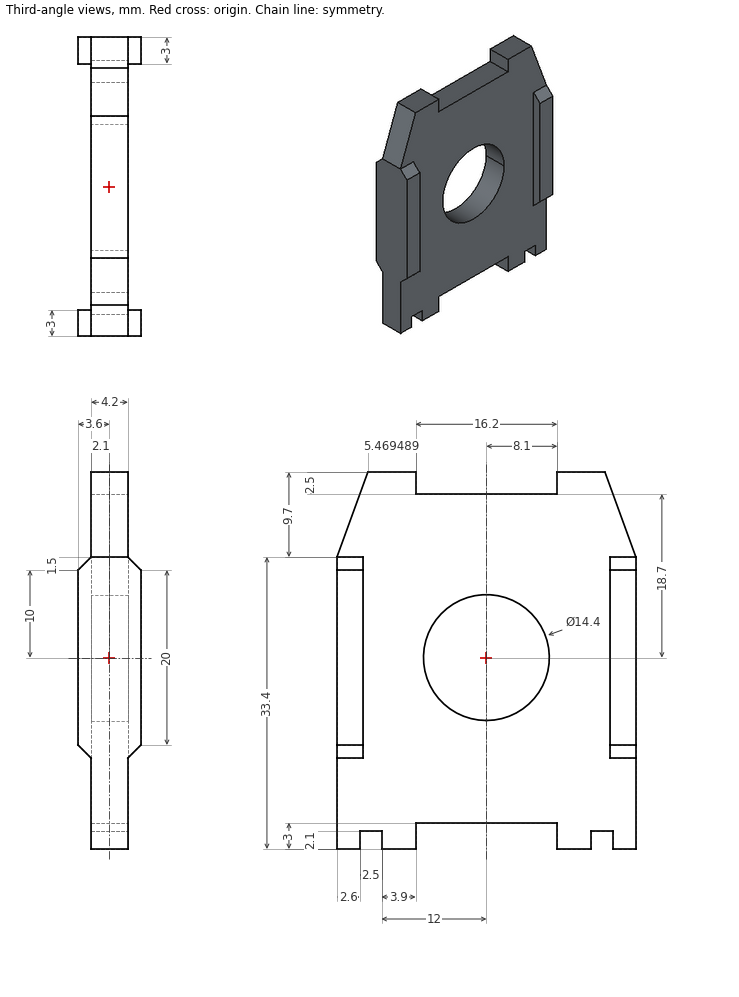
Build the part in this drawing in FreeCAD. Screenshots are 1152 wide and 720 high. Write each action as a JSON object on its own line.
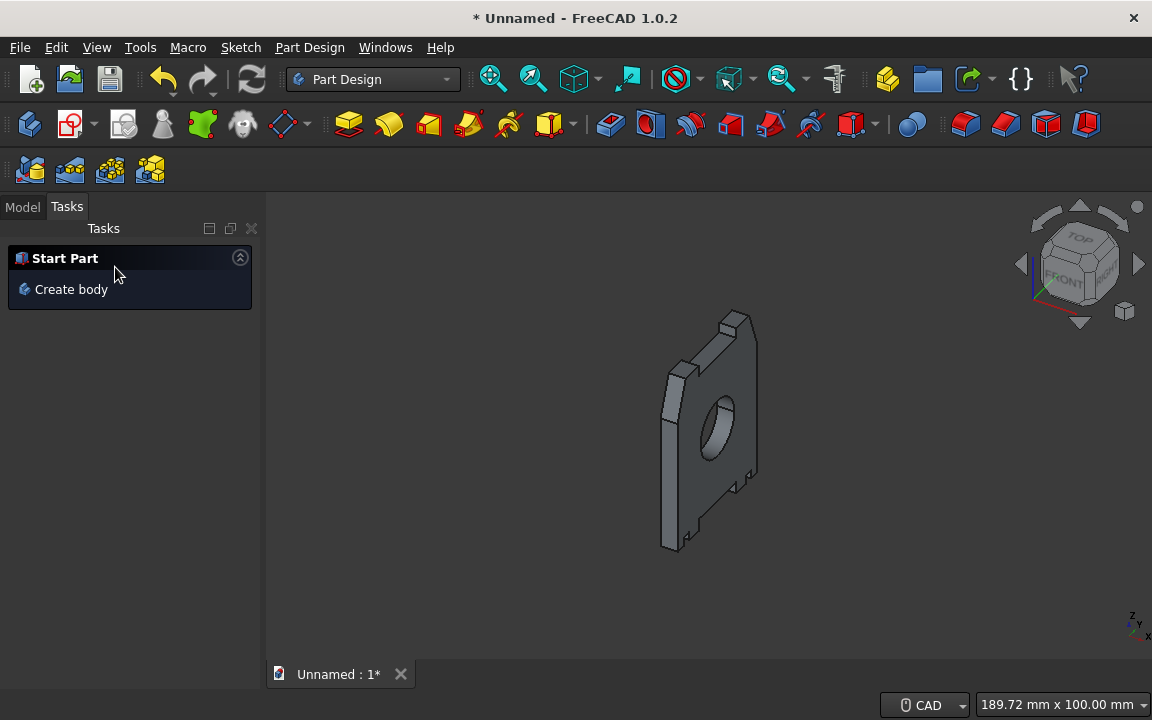
{"action": "key", "text": "4"}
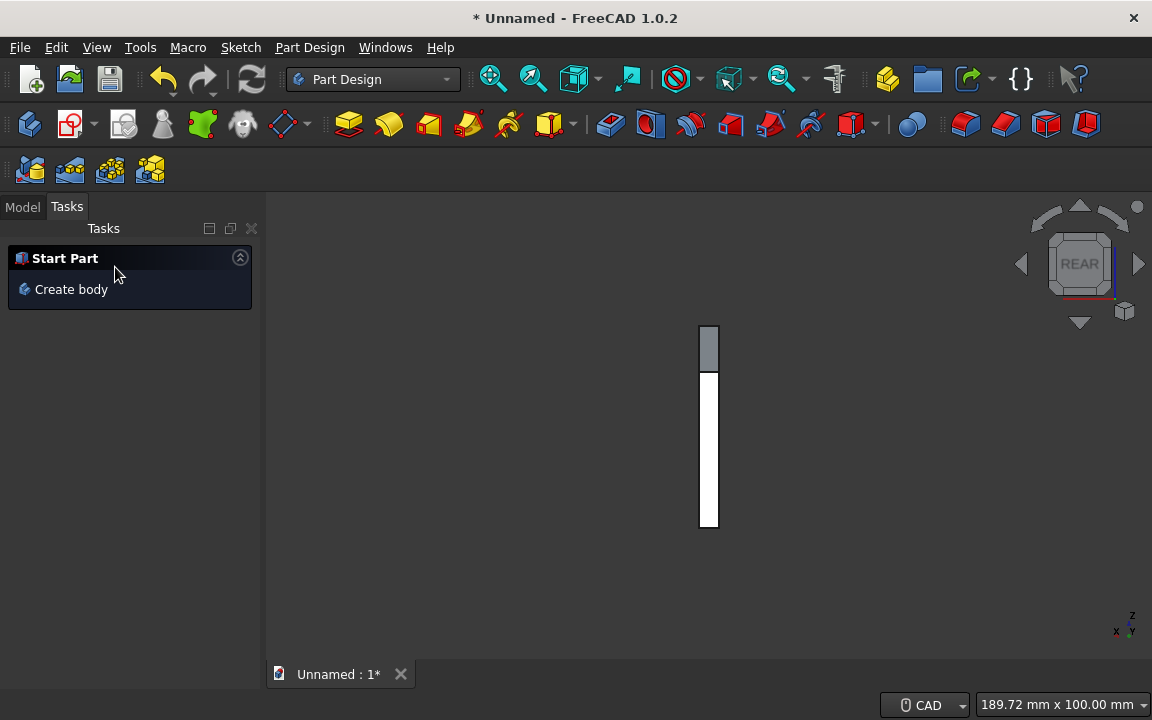
{"action": "key", "text": "v f"}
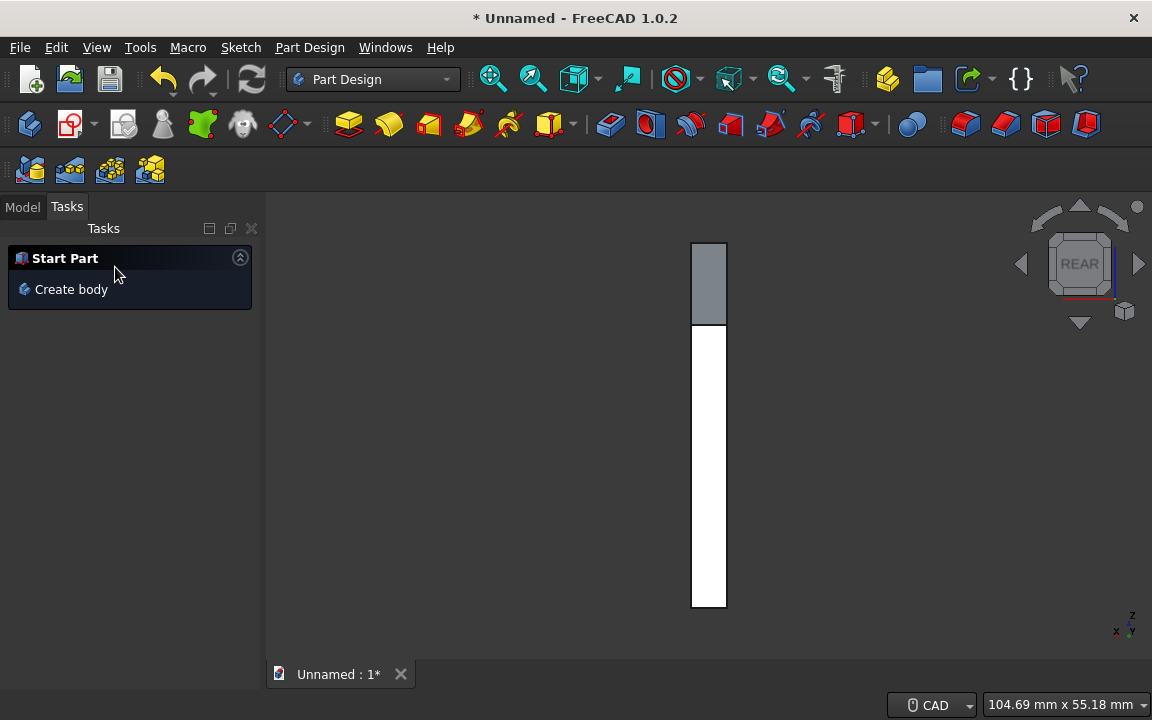
{"action": "left_click", "coordinate": [709, 546]}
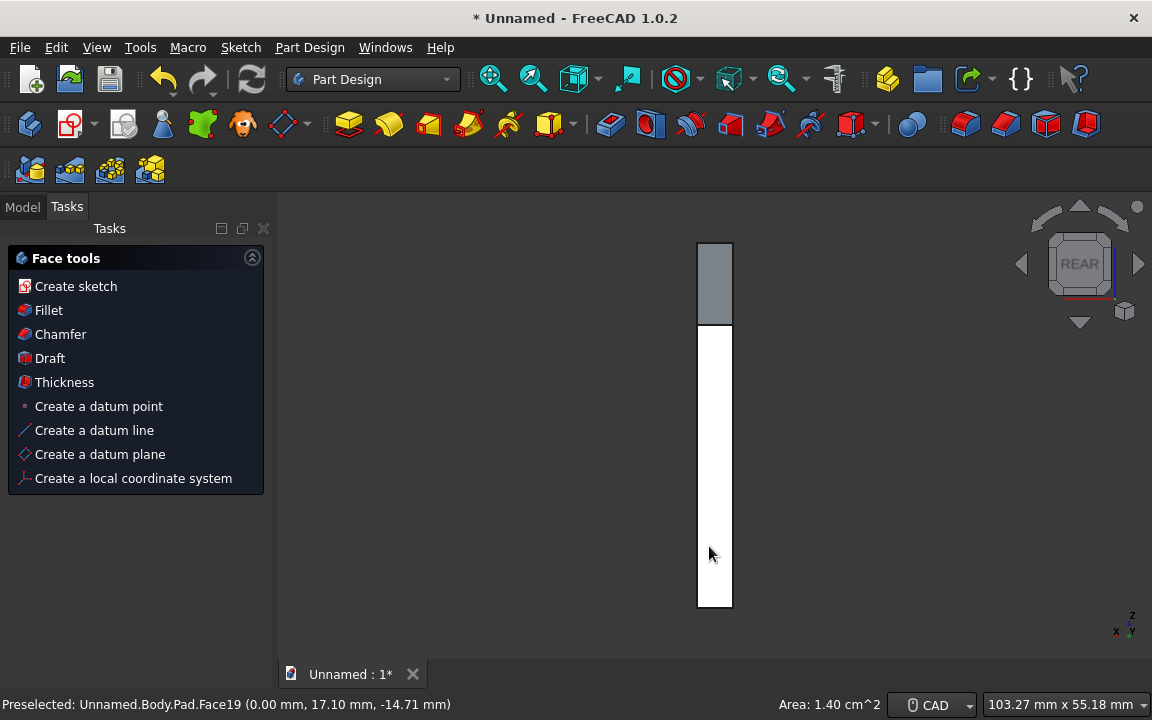
{"action": "left_click", "coordinate": [70, 124]}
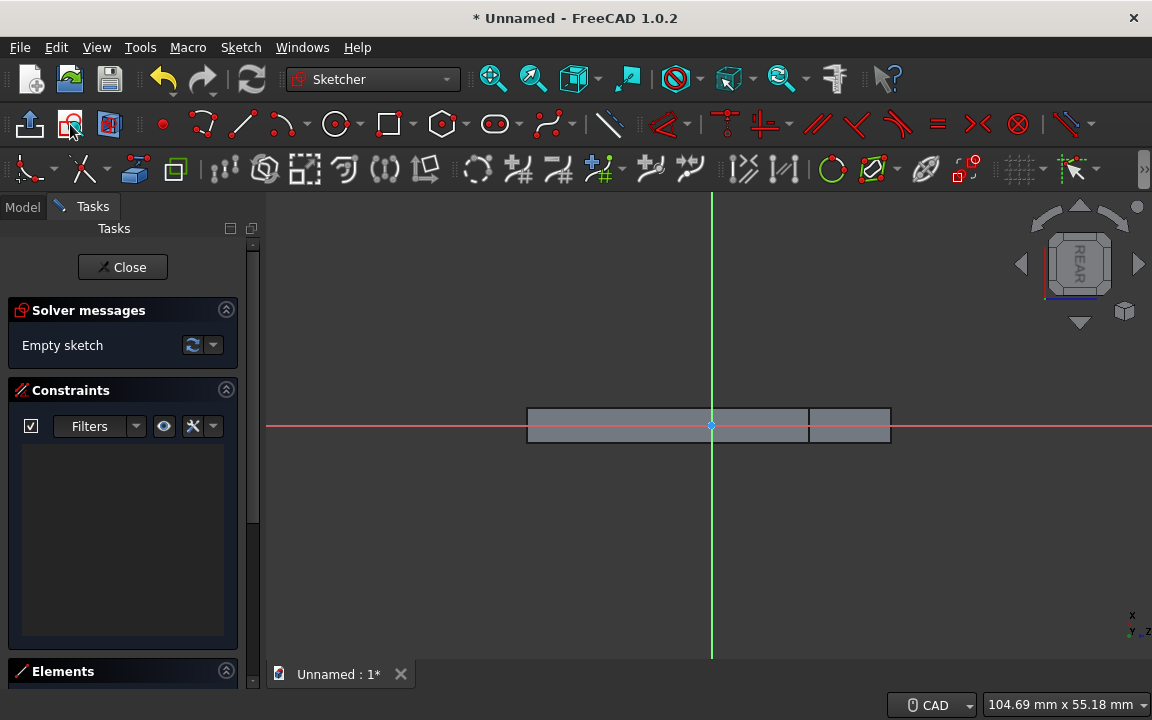
{"action": "scroll", "coordinate": [754, 425], "scroll_direction": "up", "scroll_amount": 5}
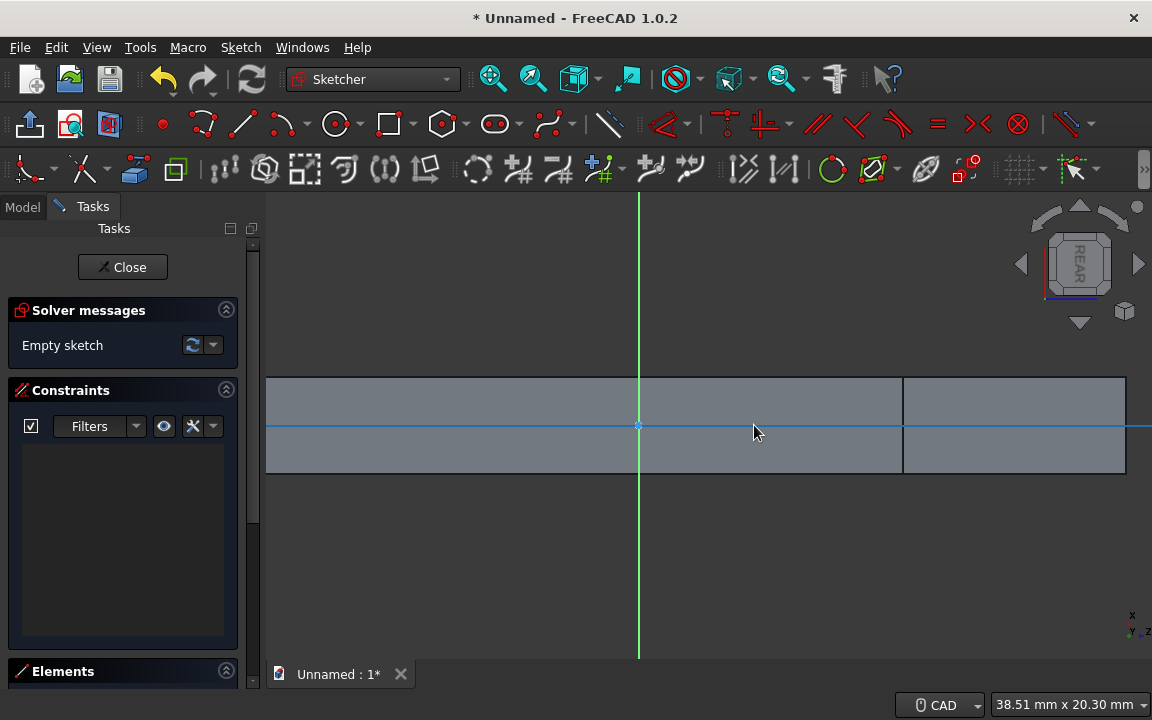
{"action": "key", "text": "g m"}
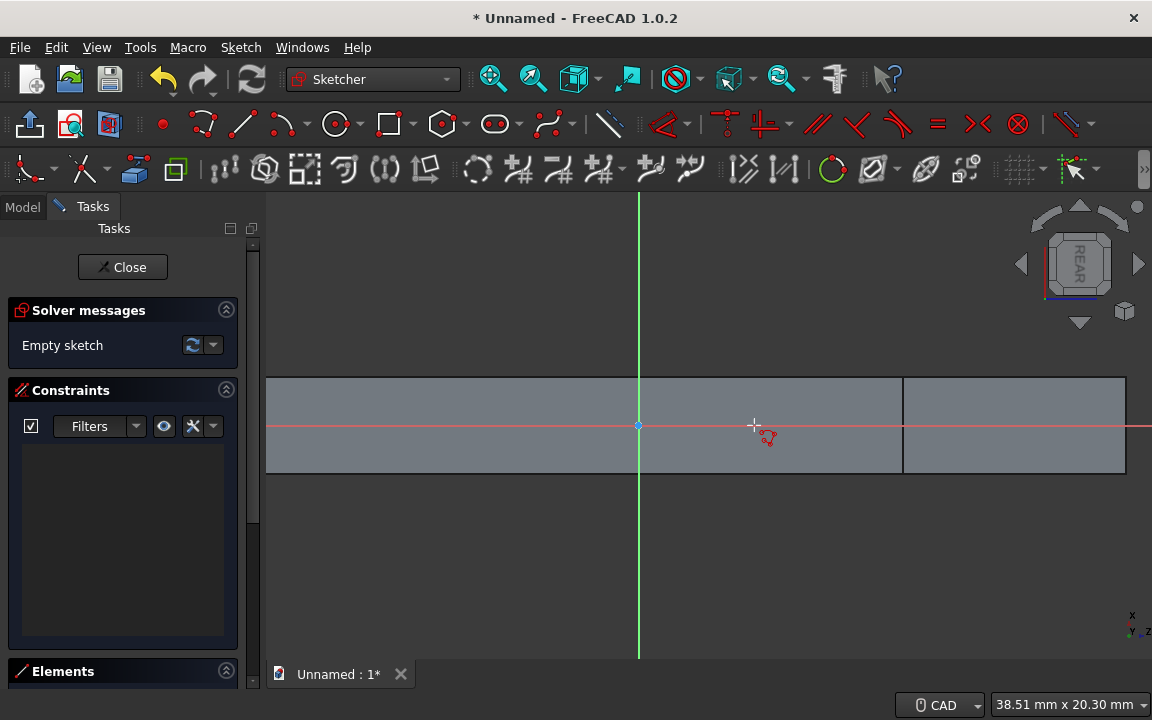
{"action": "left_click", "coordinate": [869, 508]}
{"action": "left_click", "coordinate": [903, 474]}
{"action": "left_click", "coordinate": [903, 377]}
{"action": "left_click", "coordinate": [869, 343]}
{"action": "left_click", "coordinate": [409, 343]}
{"action": "left_click", "coordinate": [374, 377]}
{"action": "left_click", "coordinate": [374, 474]}
{"action": "left_click", "coordinate": [409, 508]}
{"action": "left_click", "coordinate": [869, 509]}
{"action": "key", "text": "Escape"}
{"action": "key", "text": "Escape"}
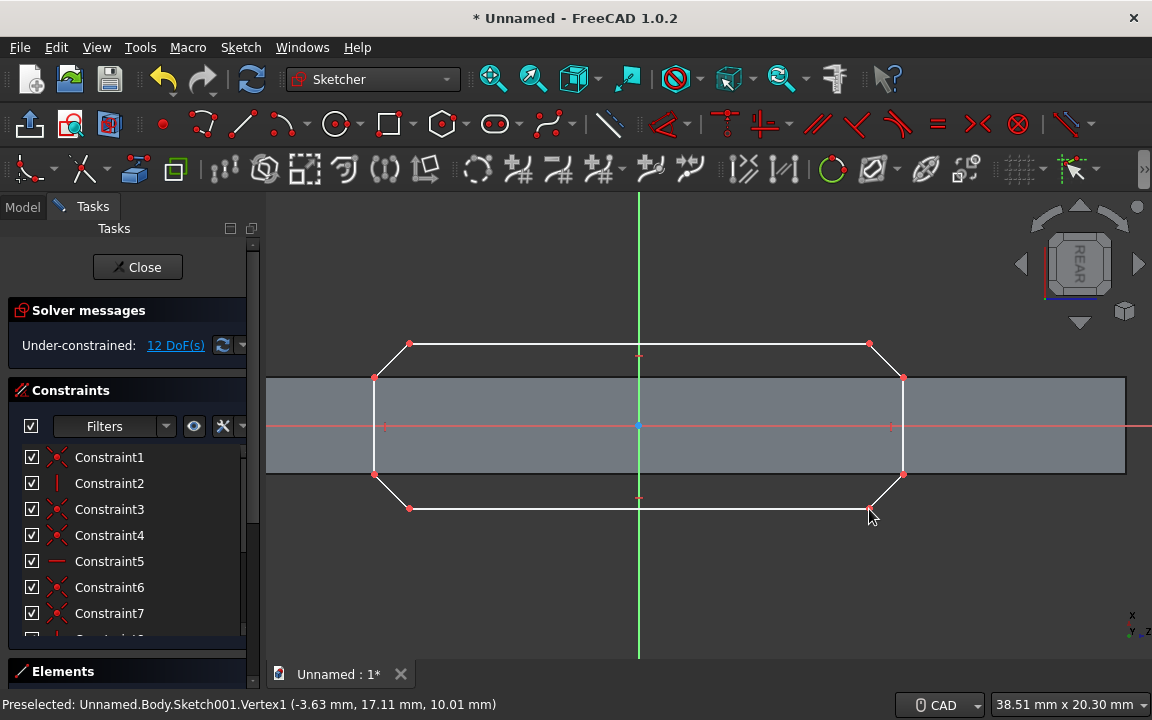
{"action": "left_click", "coordinate": [869, 509]}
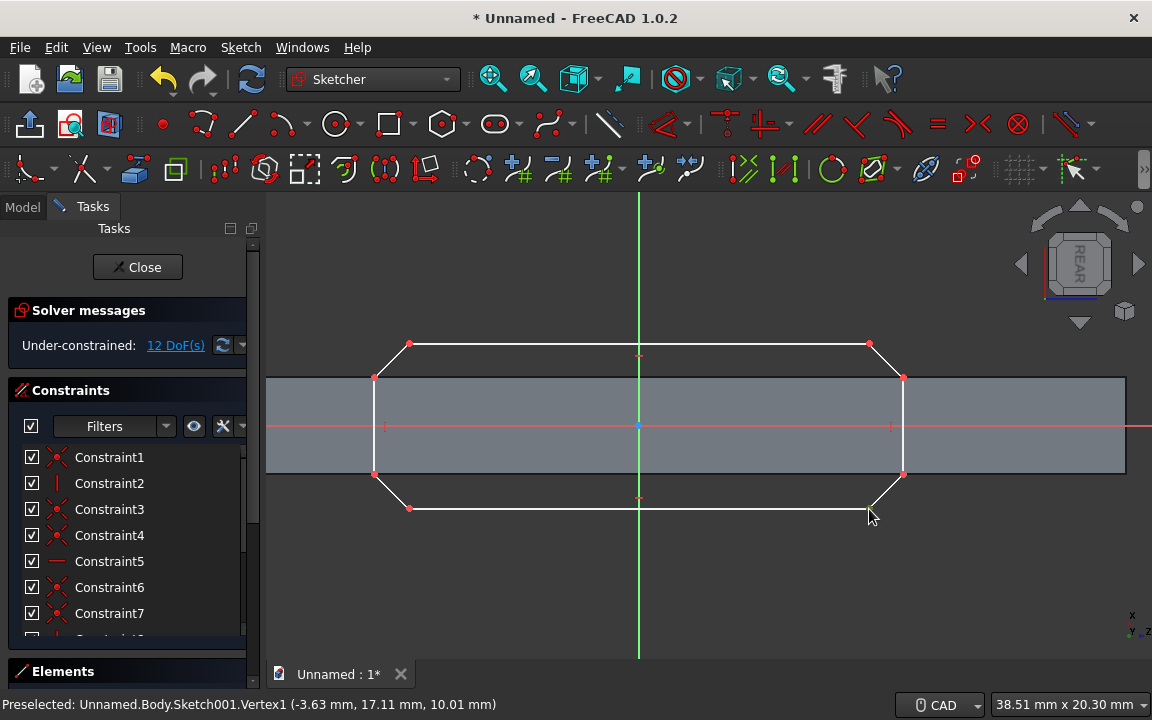
{"action": "left_click", "coordinate": [869, 344]}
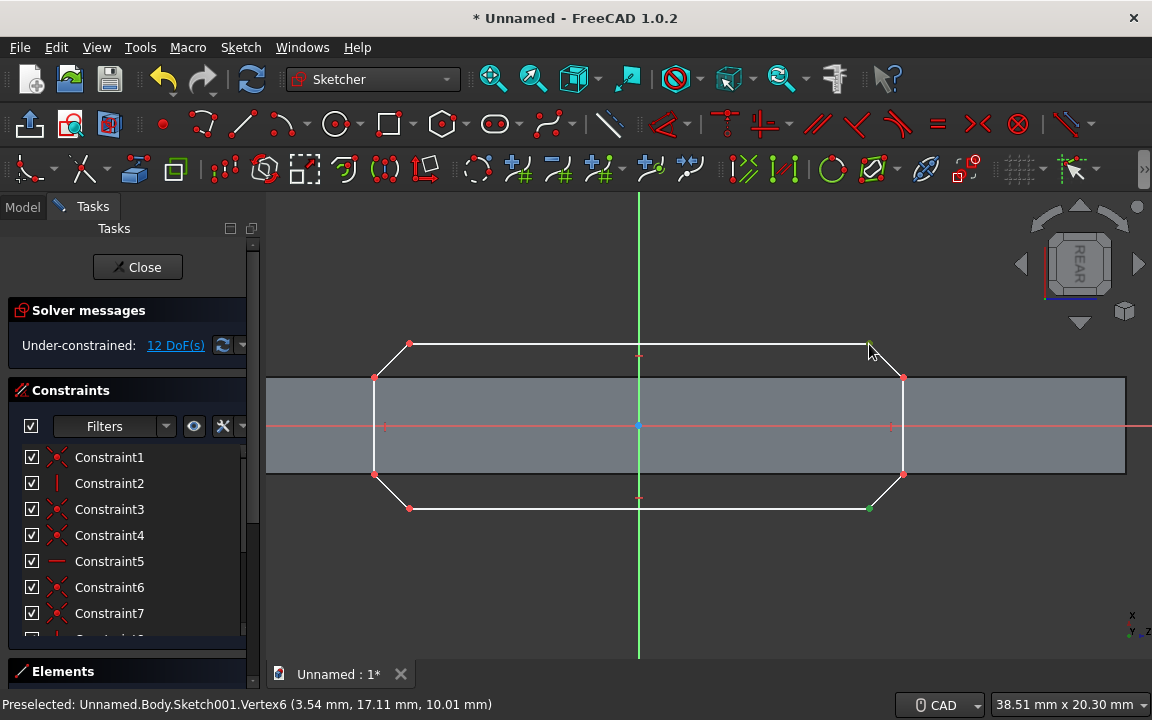
{"action": "left_click", "coordinate": [344, 425]}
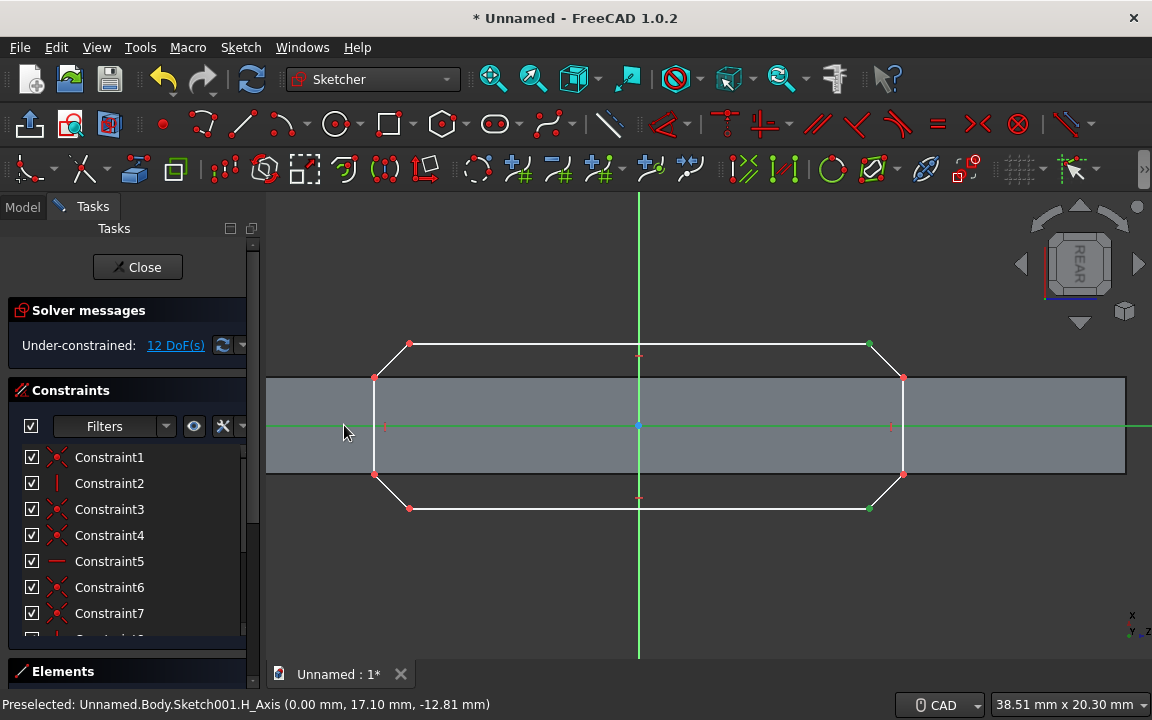
{"action": "left_click", "coordinate": [978, 124]}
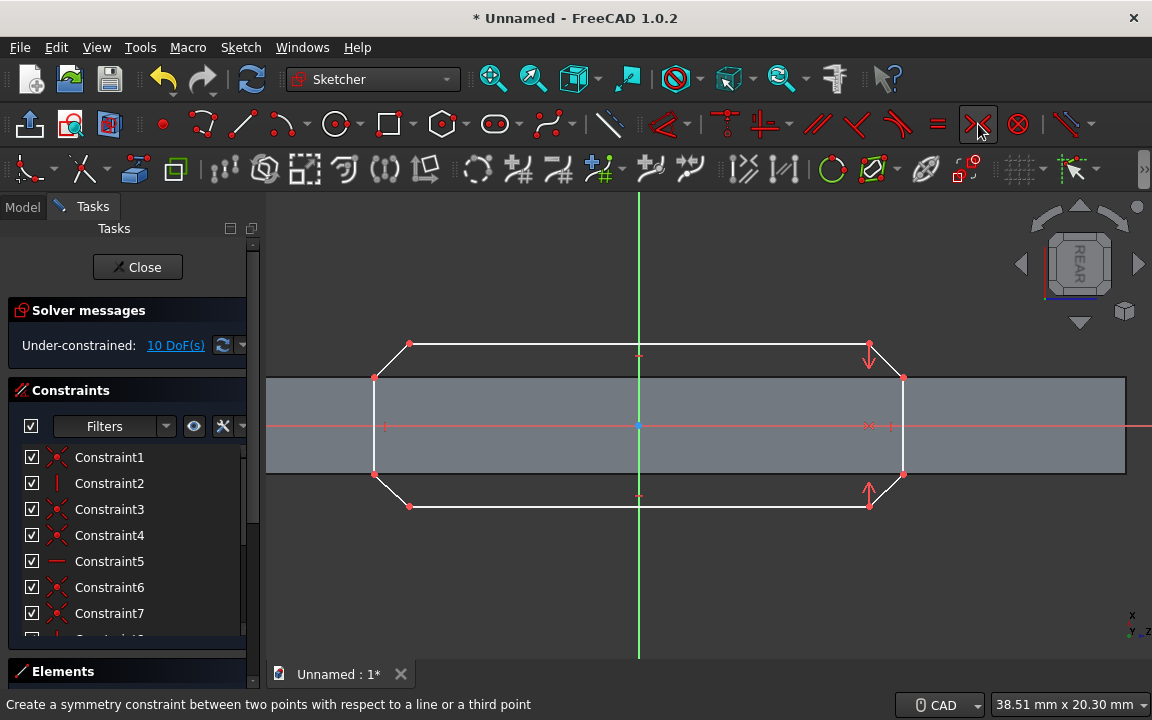
{"action": "left_click", "coordinate": [903, 378]}